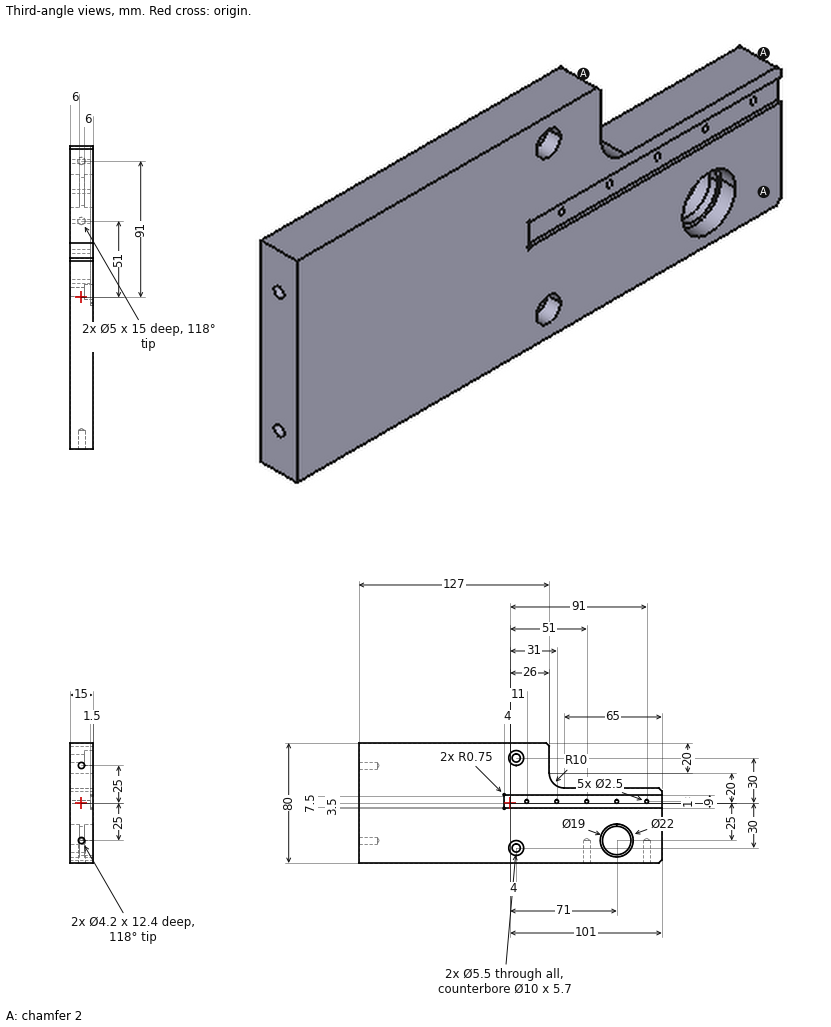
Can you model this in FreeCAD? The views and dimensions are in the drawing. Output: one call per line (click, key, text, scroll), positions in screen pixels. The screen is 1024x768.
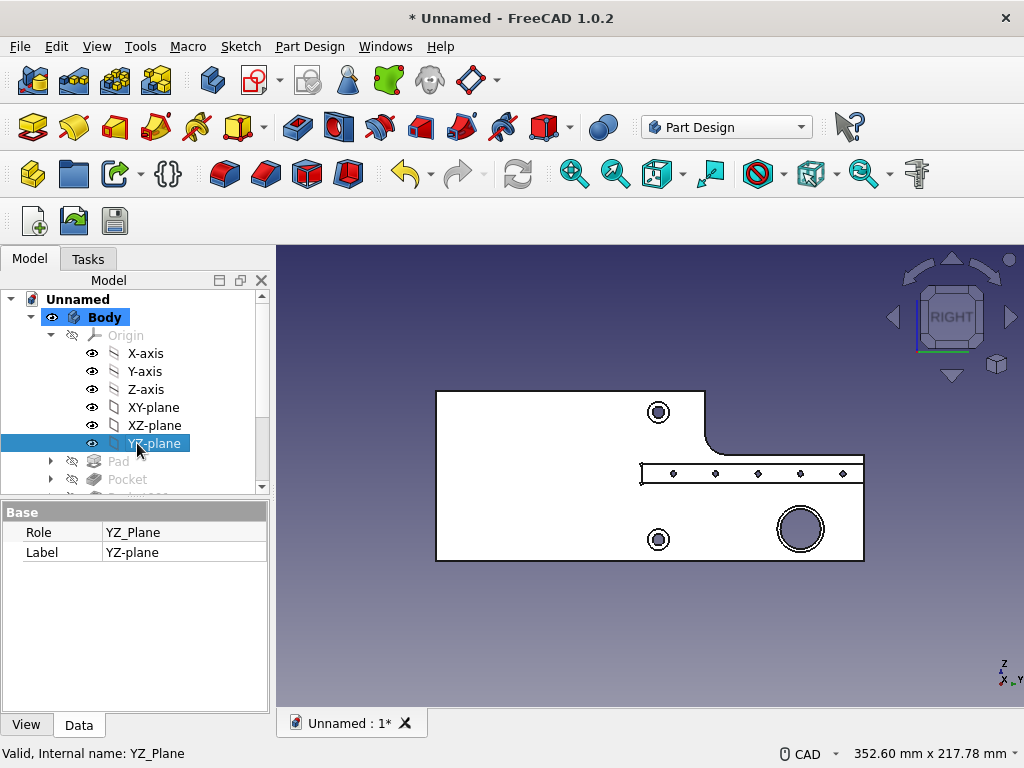
click(470, 80)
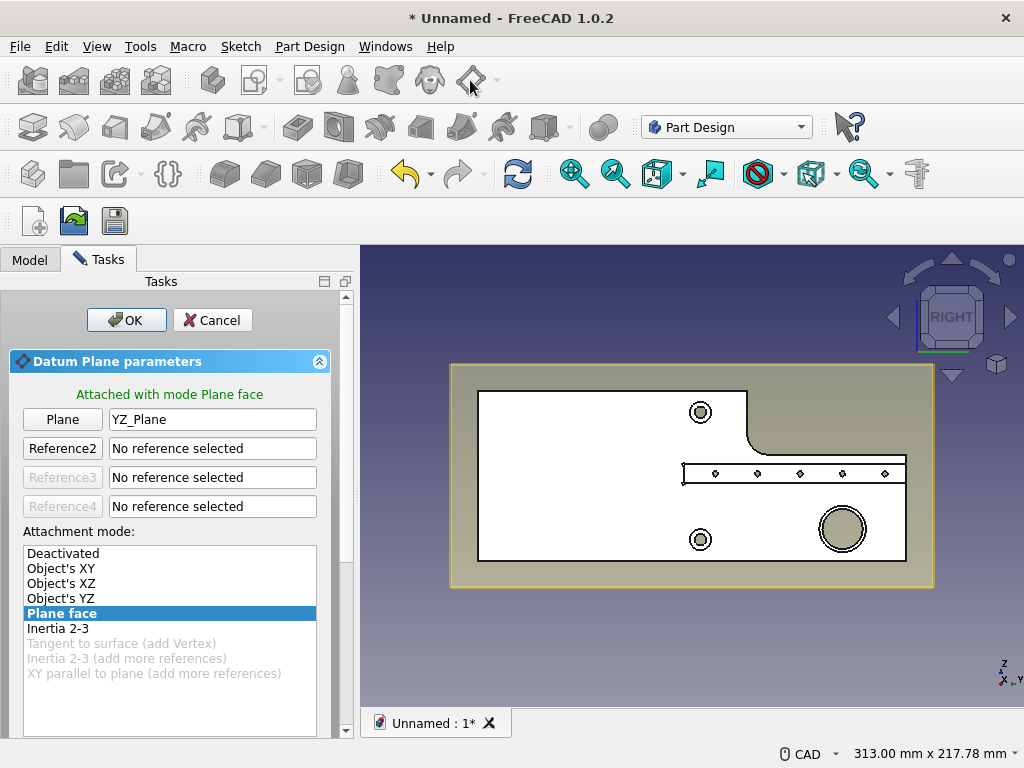
scroll(346, 514, down, 4)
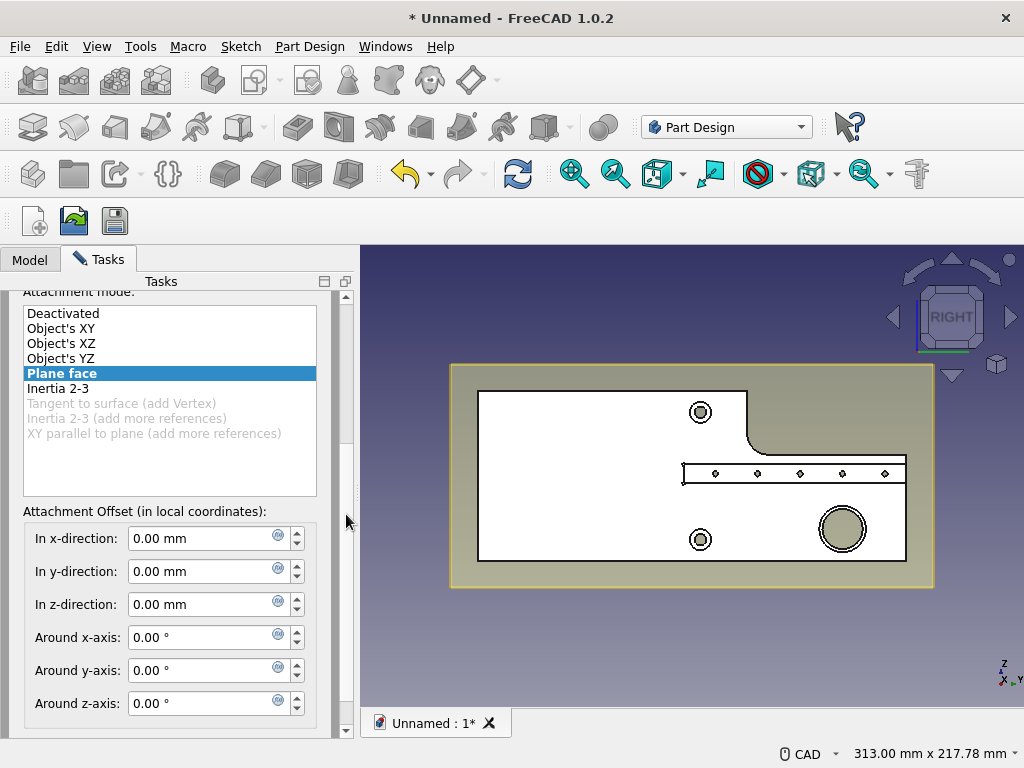
triple_click(210, 604)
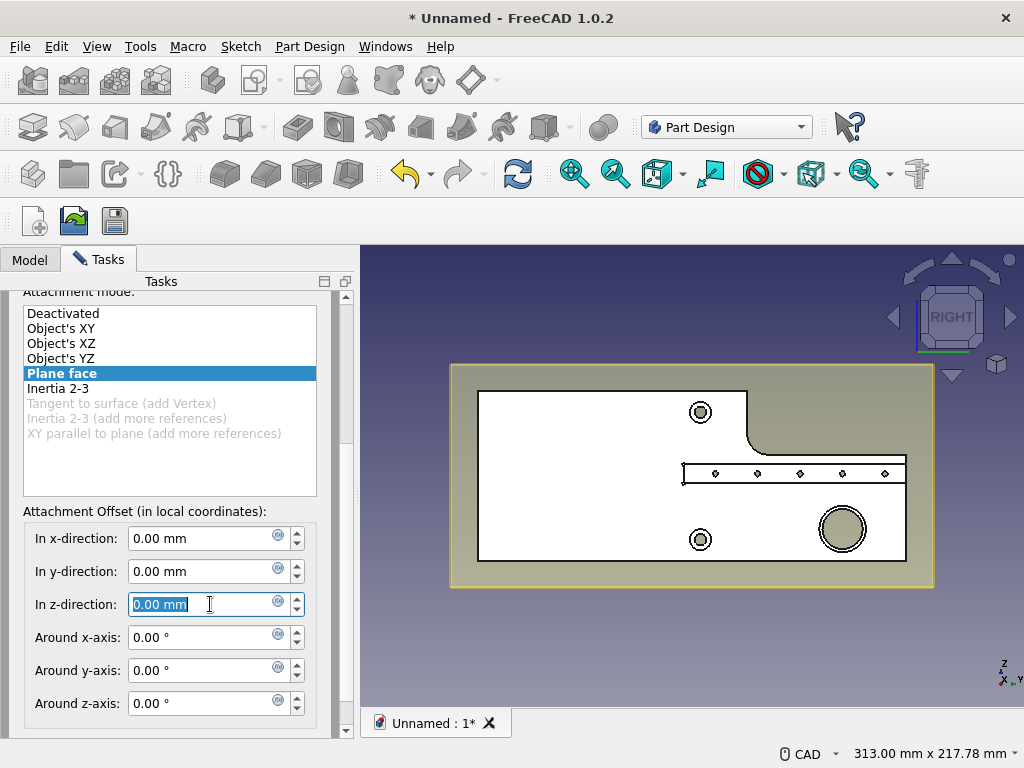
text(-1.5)
key(Tab)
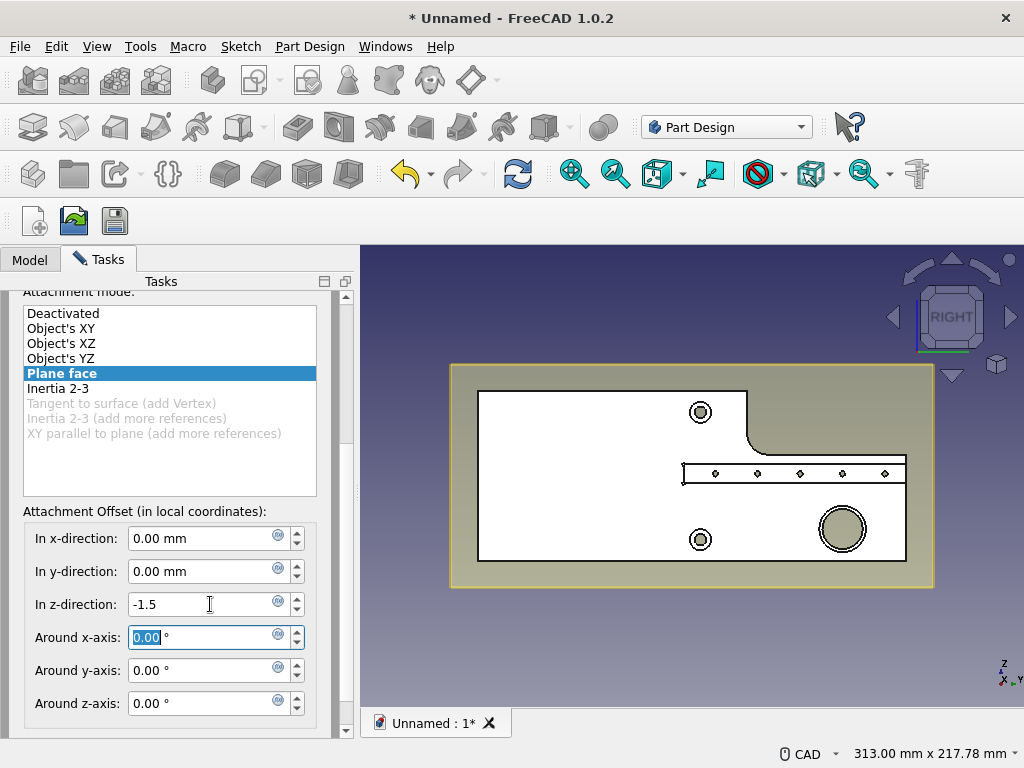
scroll(346, 514, up, 5)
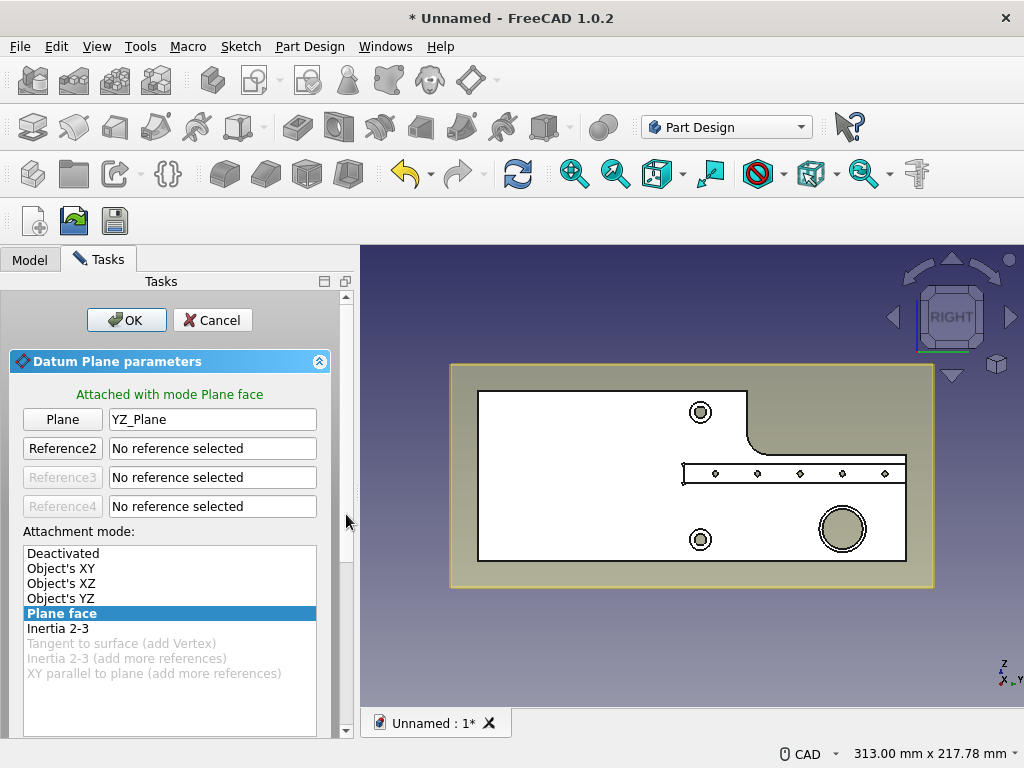
click(127, 320)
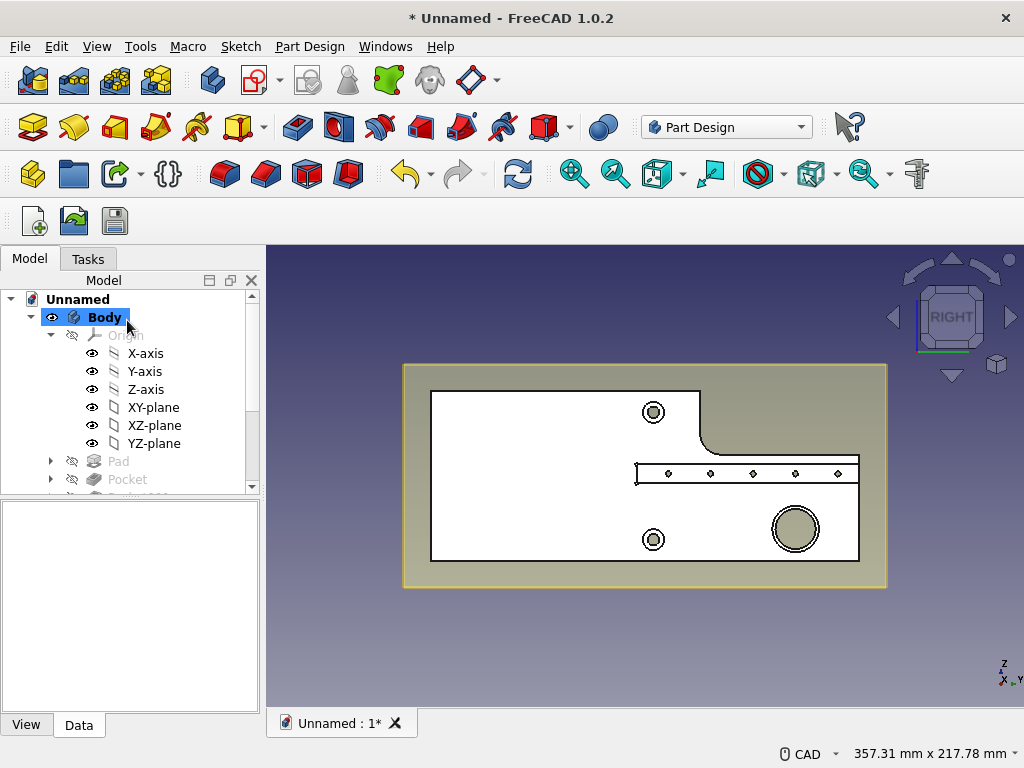
scroll(101, 385, down, 3)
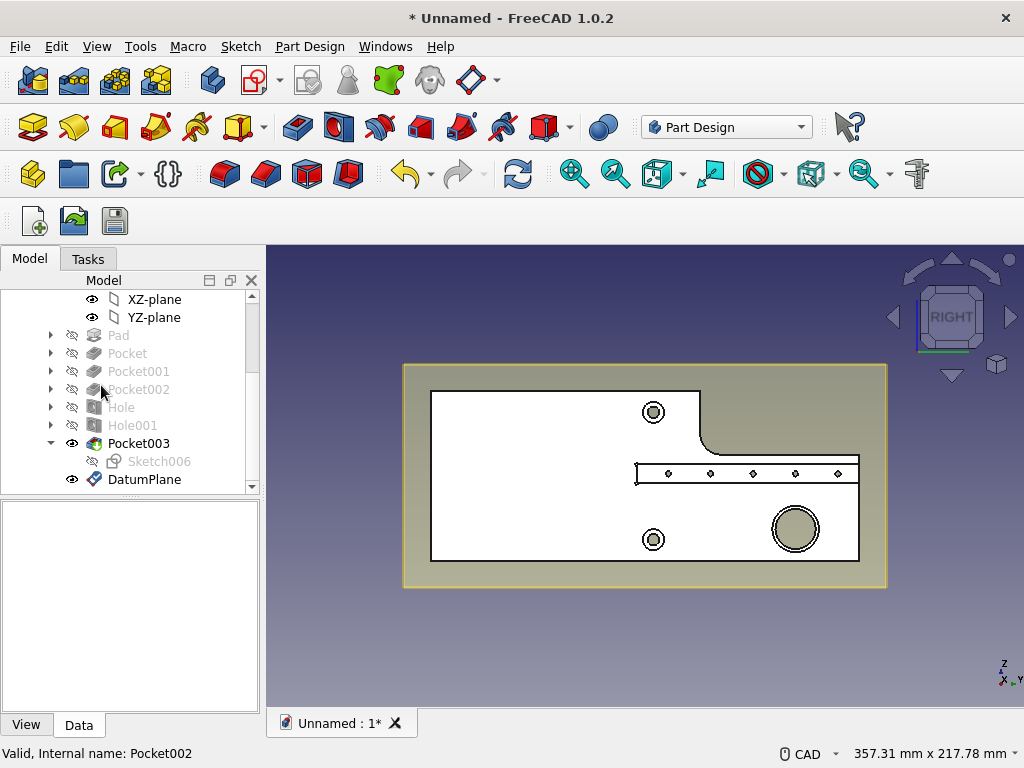
click(117, 479)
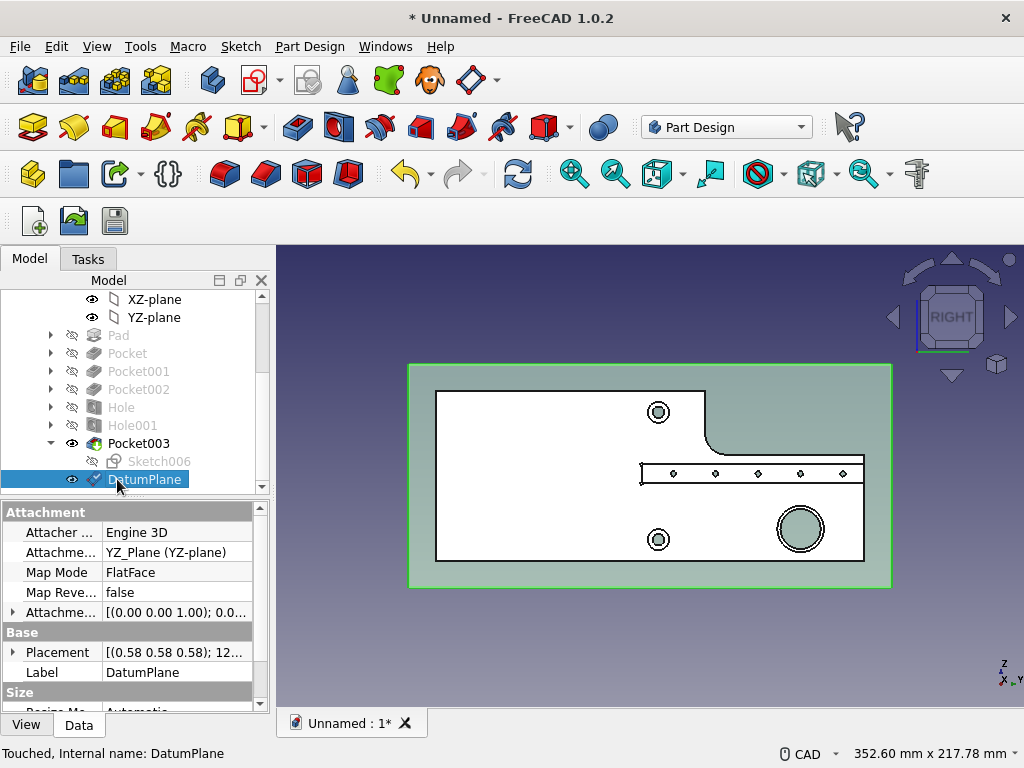
click(254, 80)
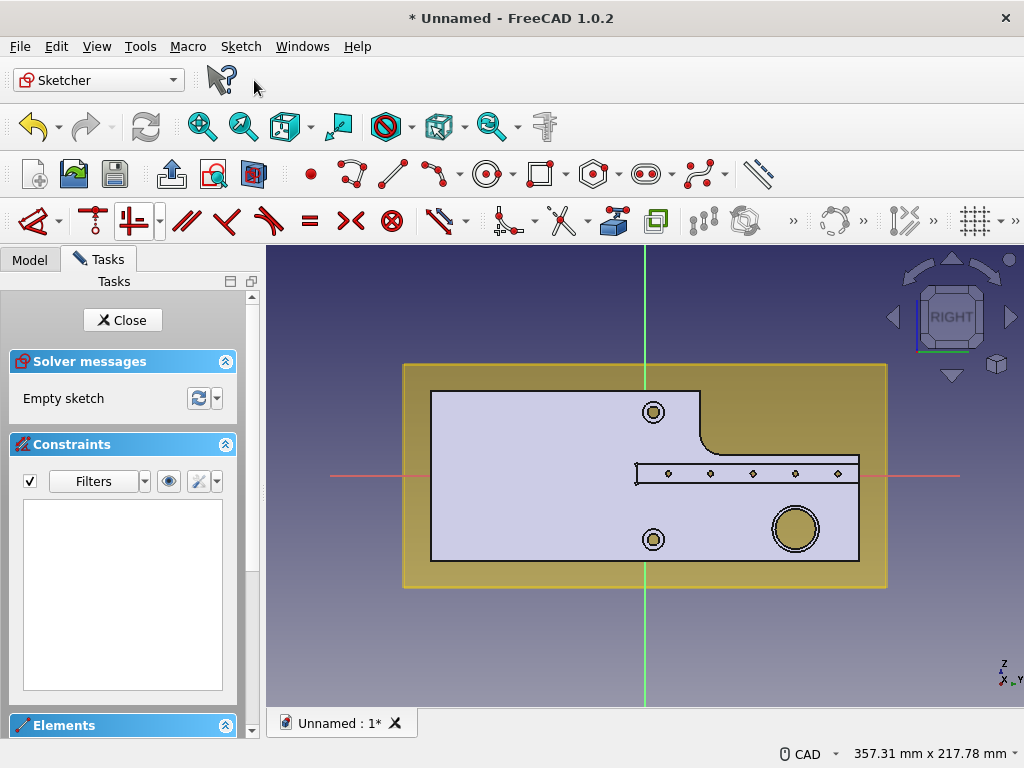
click(254, 174)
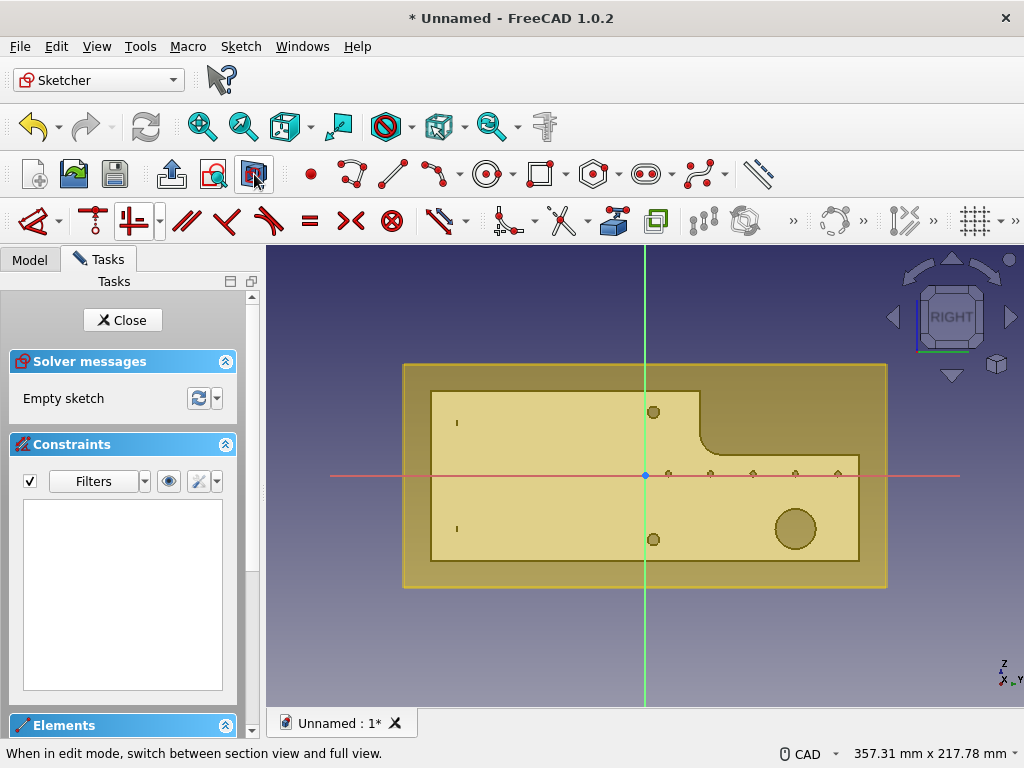
scroll(839, 540, up, 9)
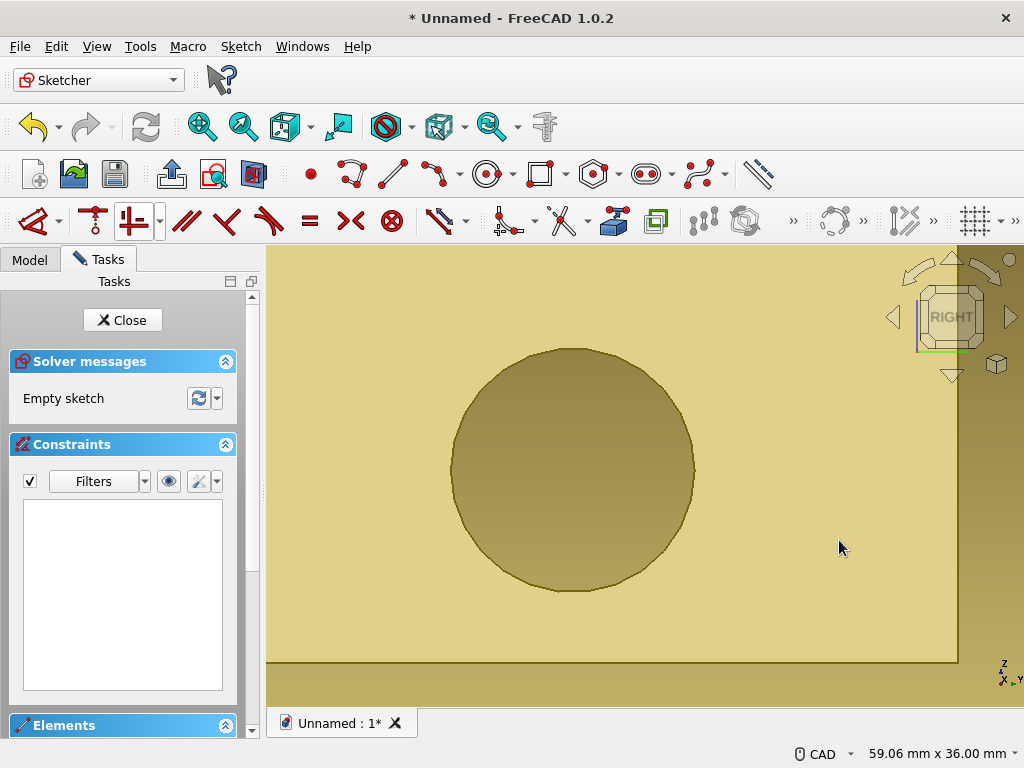
click(486, 174)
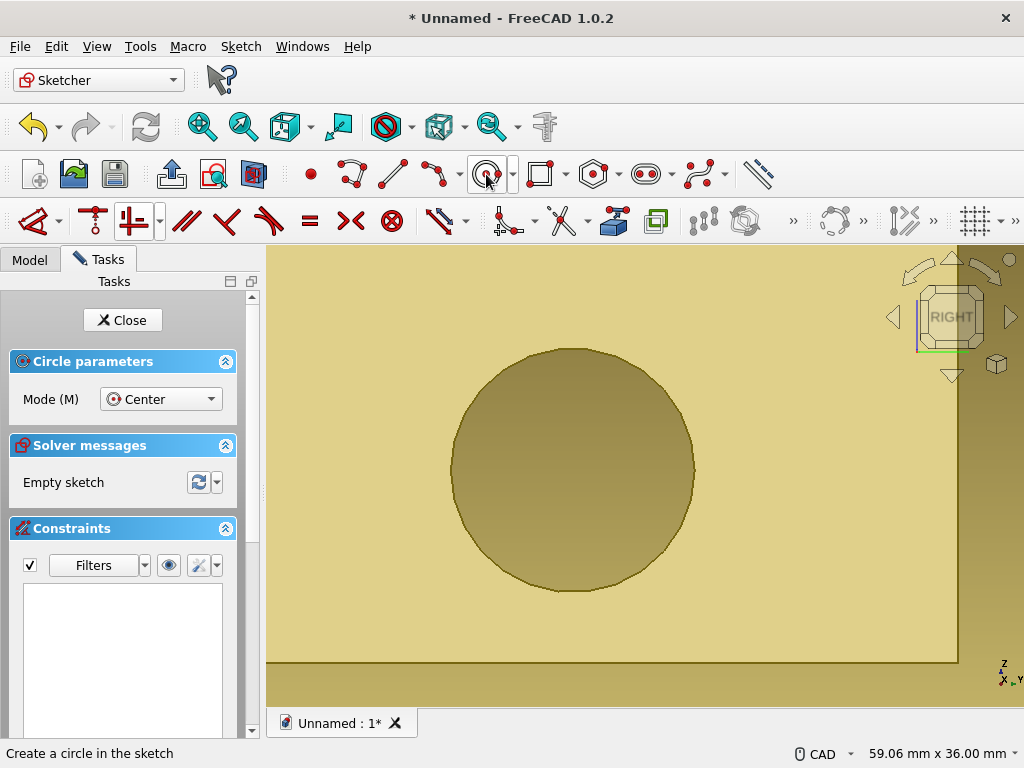
click(573, 470)
click(673, 371)
key(Escape)